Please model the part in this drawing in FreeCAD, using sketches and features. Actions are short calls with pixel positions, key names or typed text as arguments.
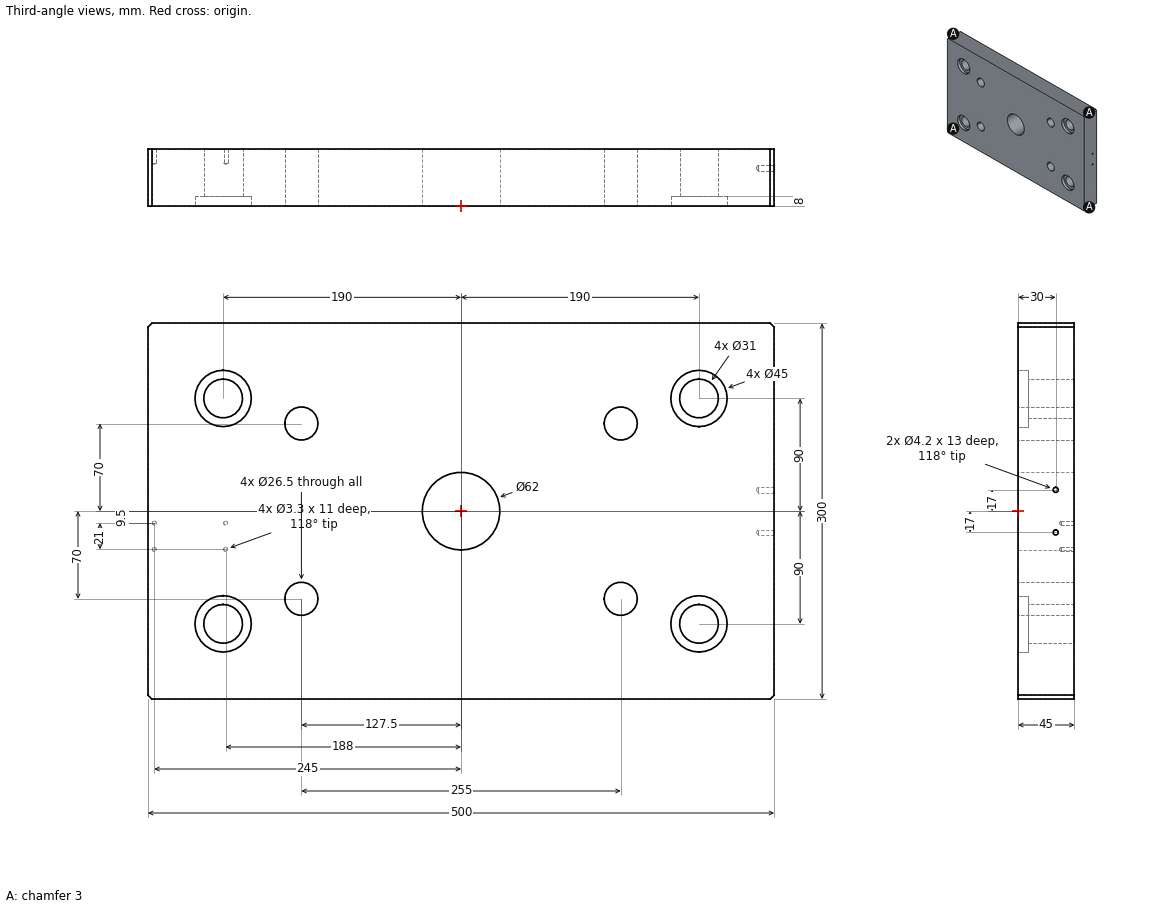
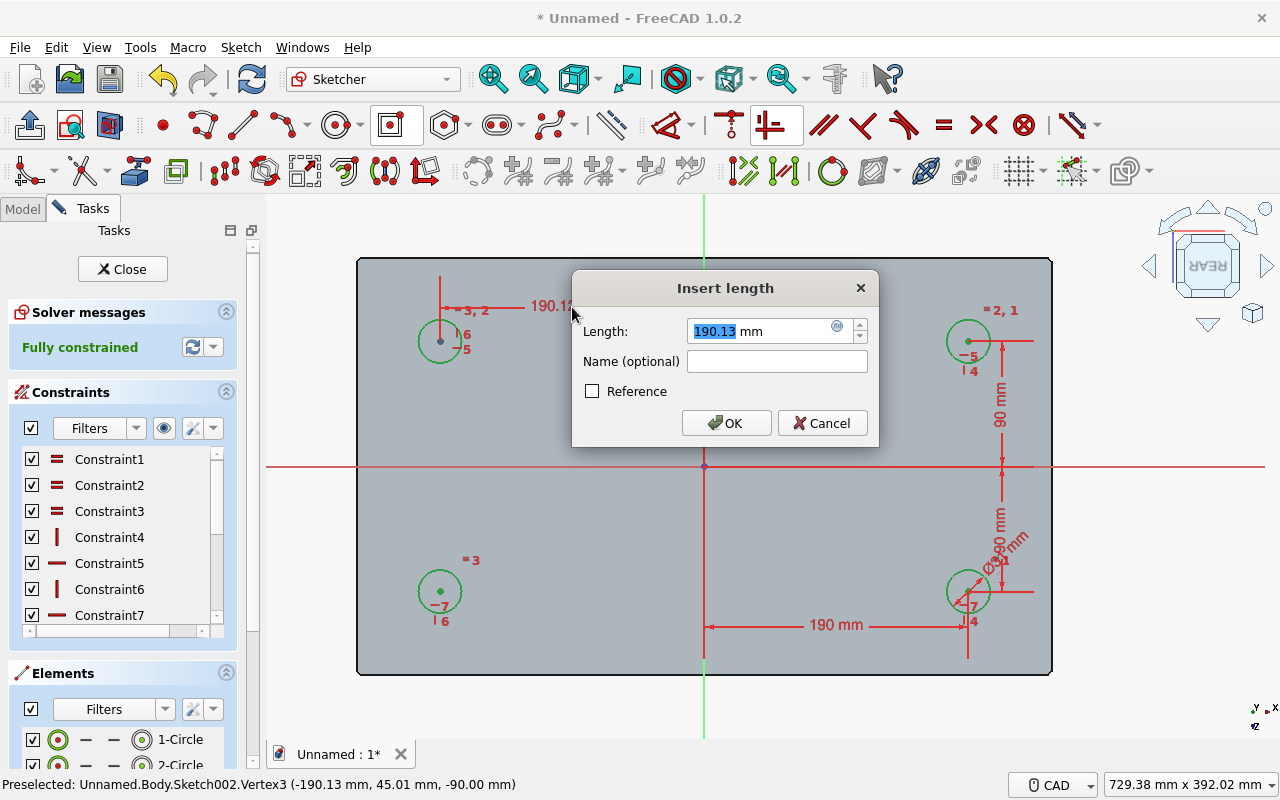
text(190)
key(Return)
key(Escape)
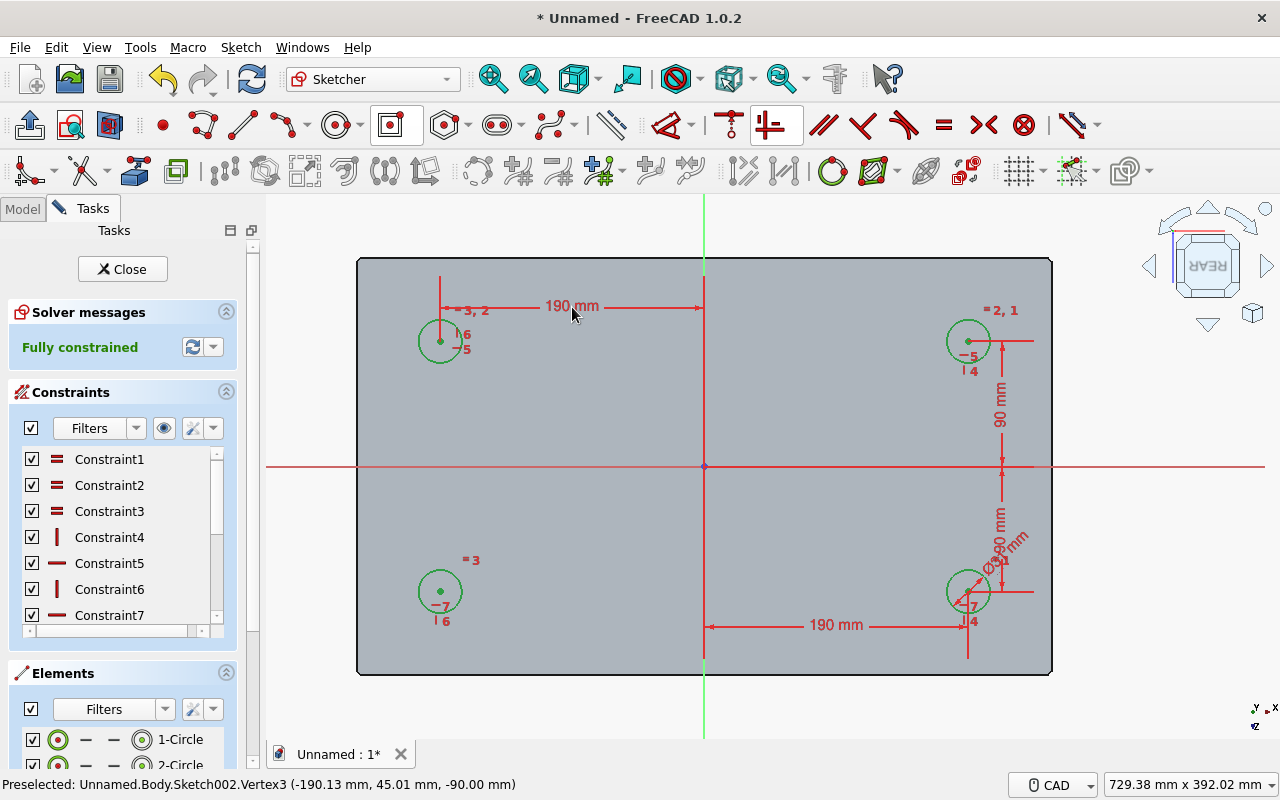
click(123, 269)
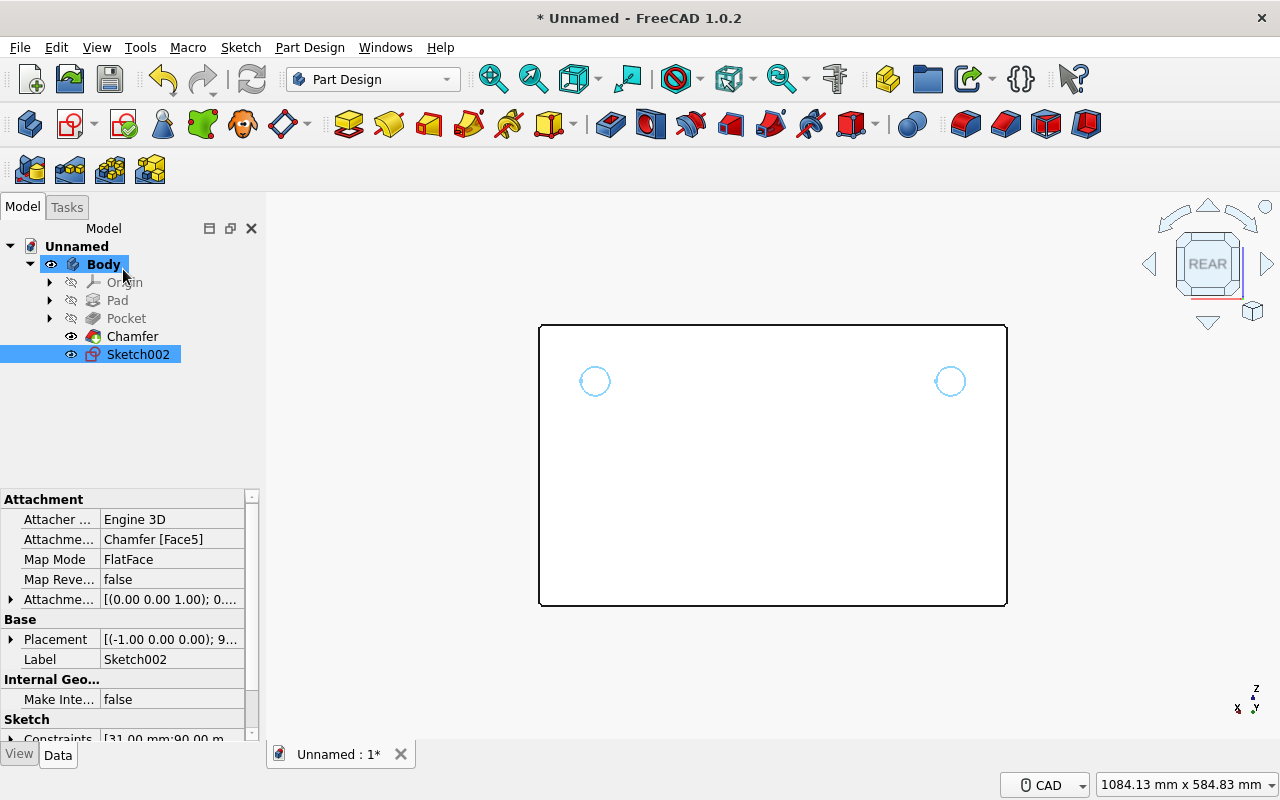
click(612, 124)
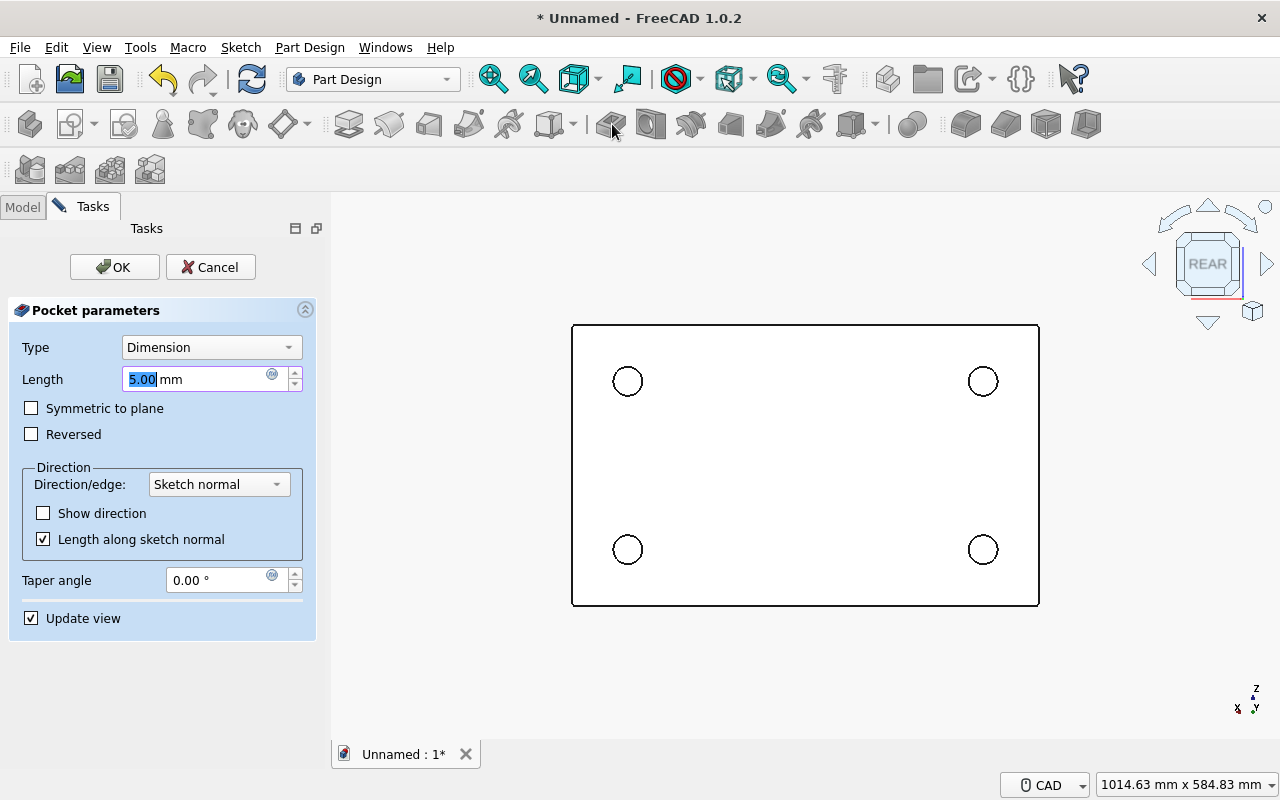
click(212, 348)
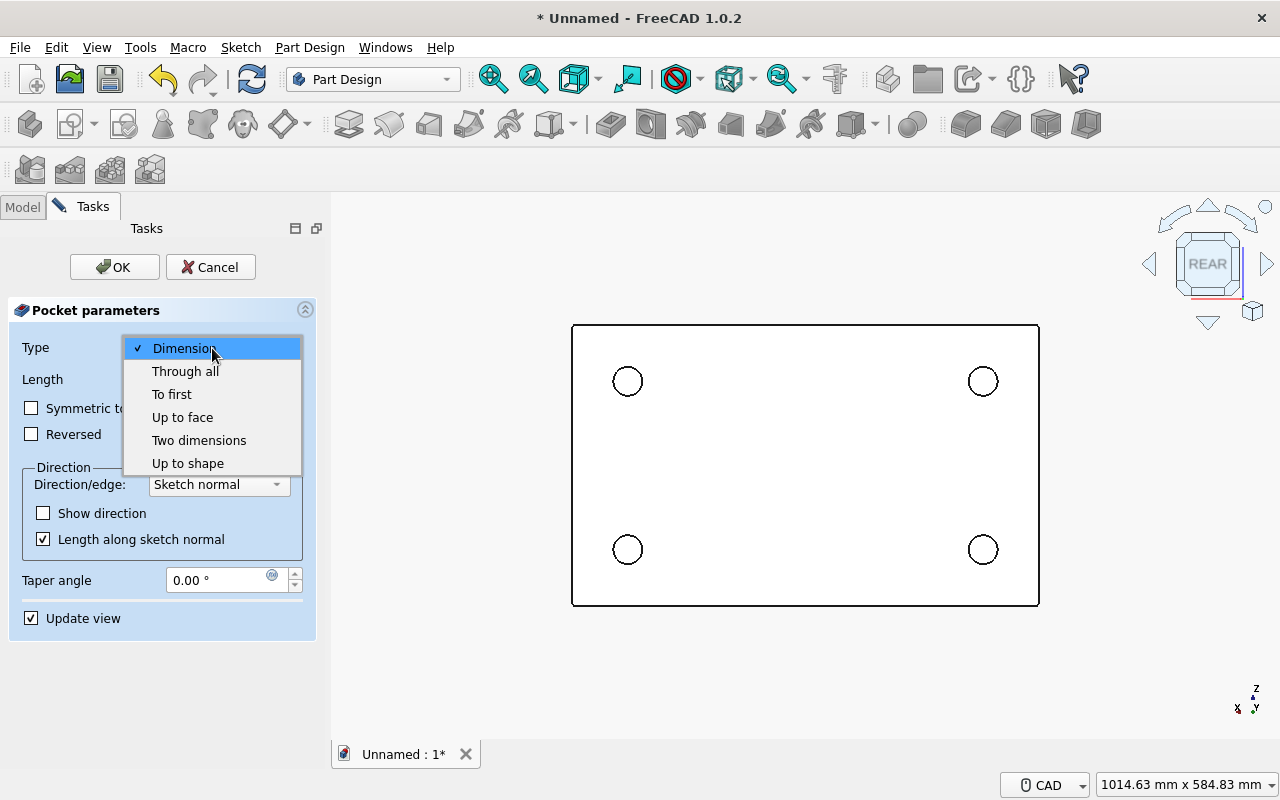
click(212, 372)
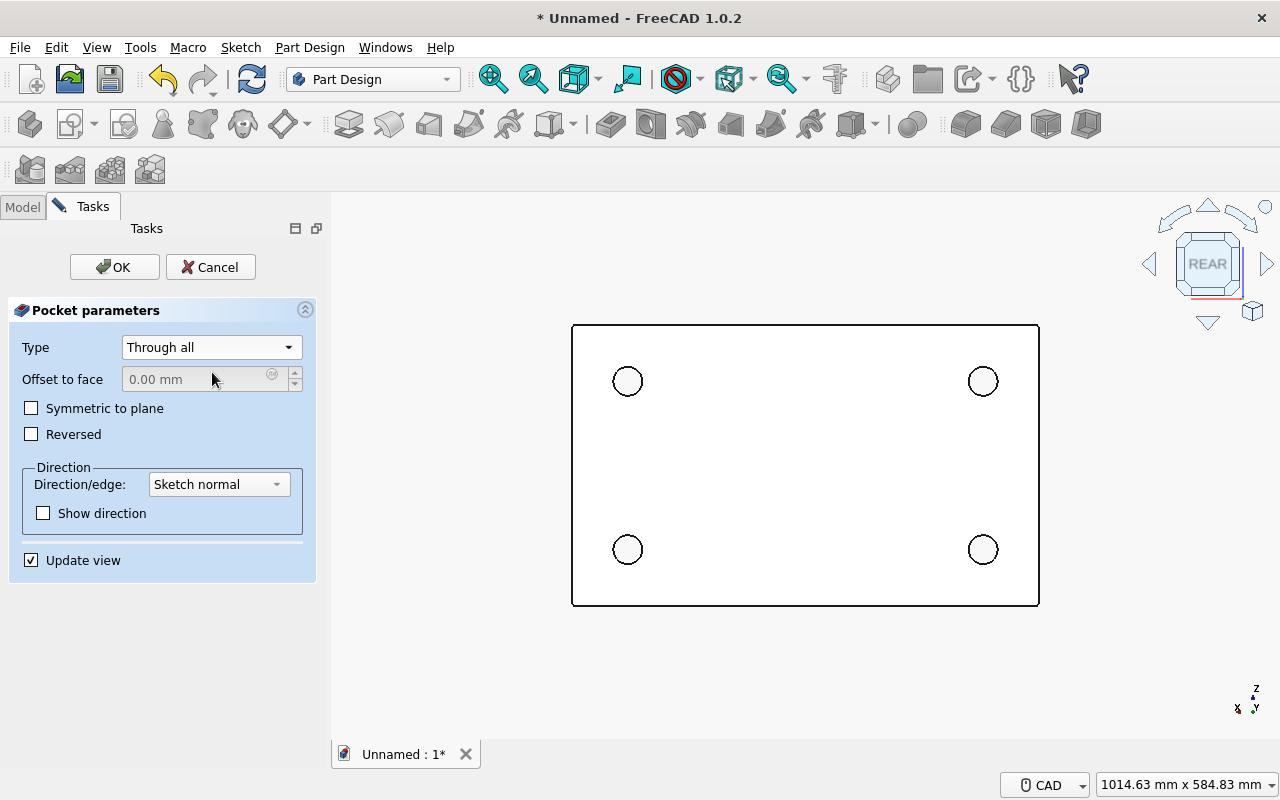
click(115, 267)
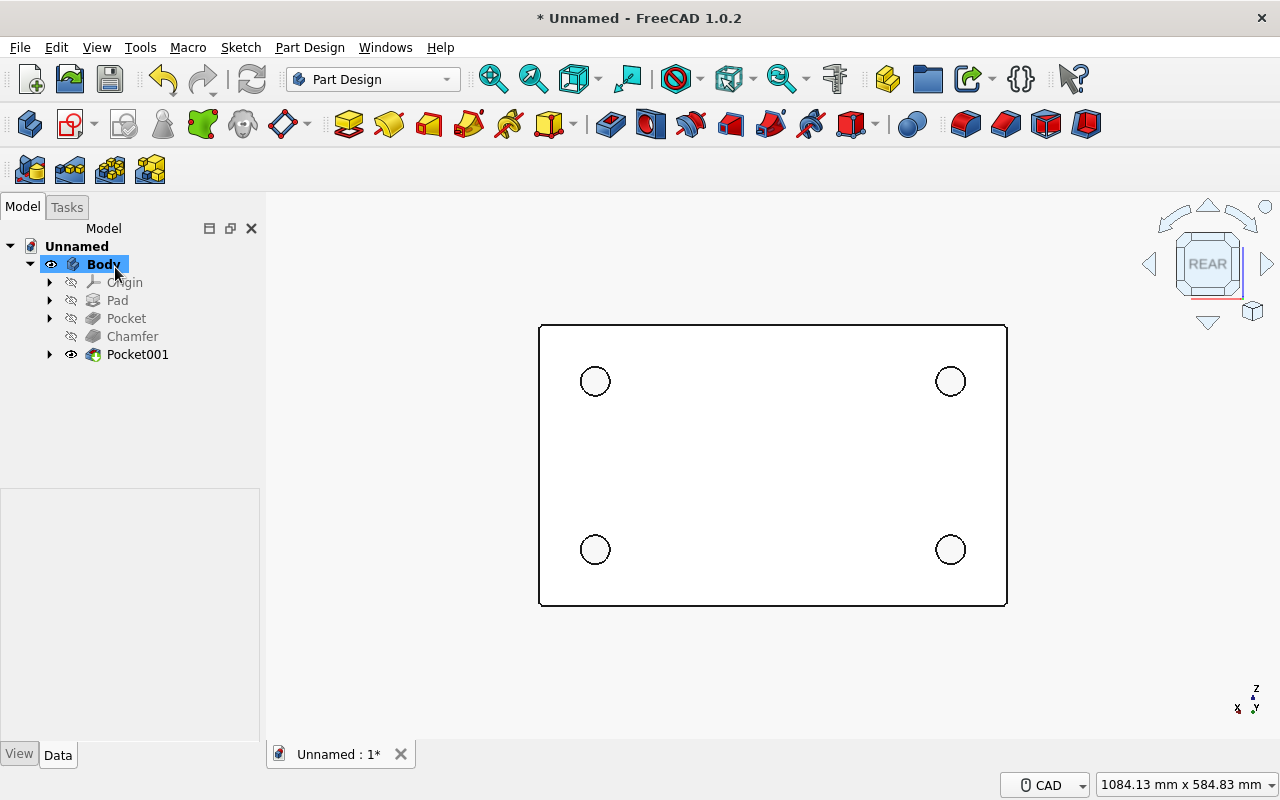
click(70, 124)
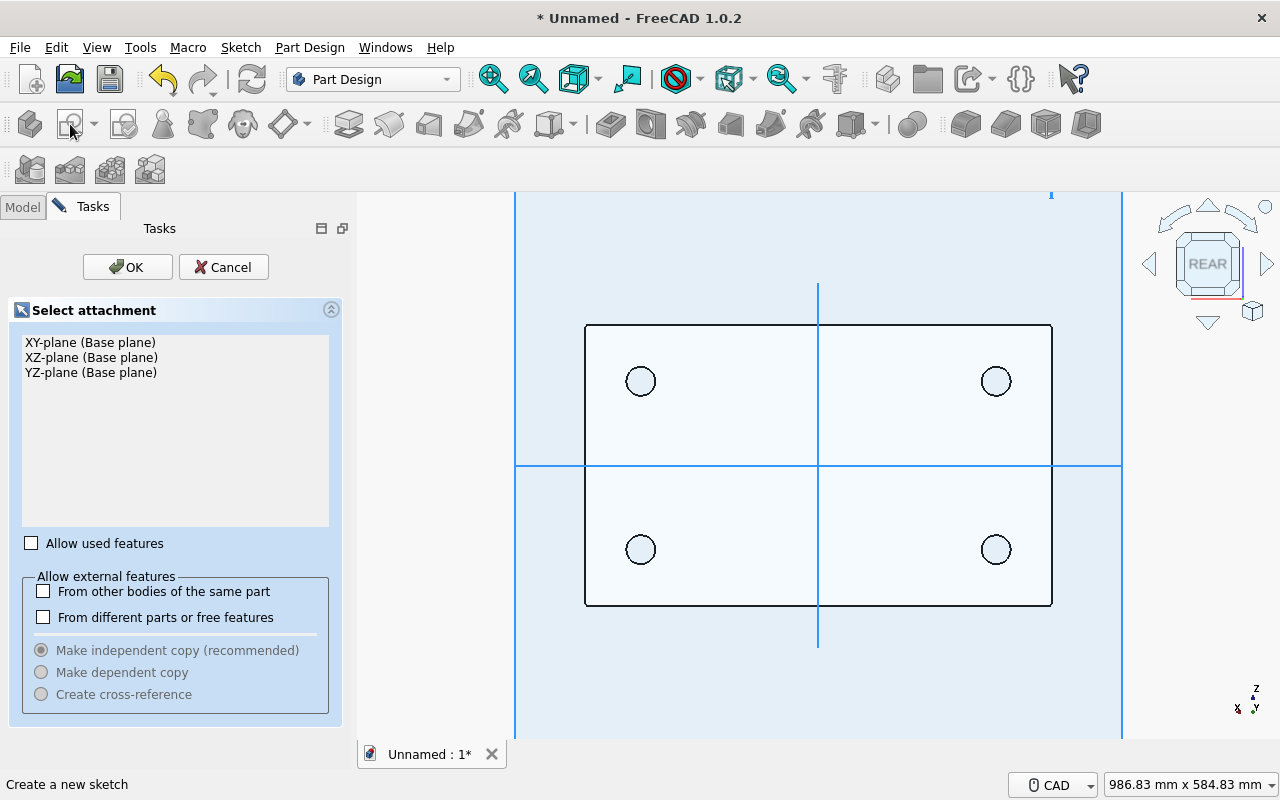
click(82, 358)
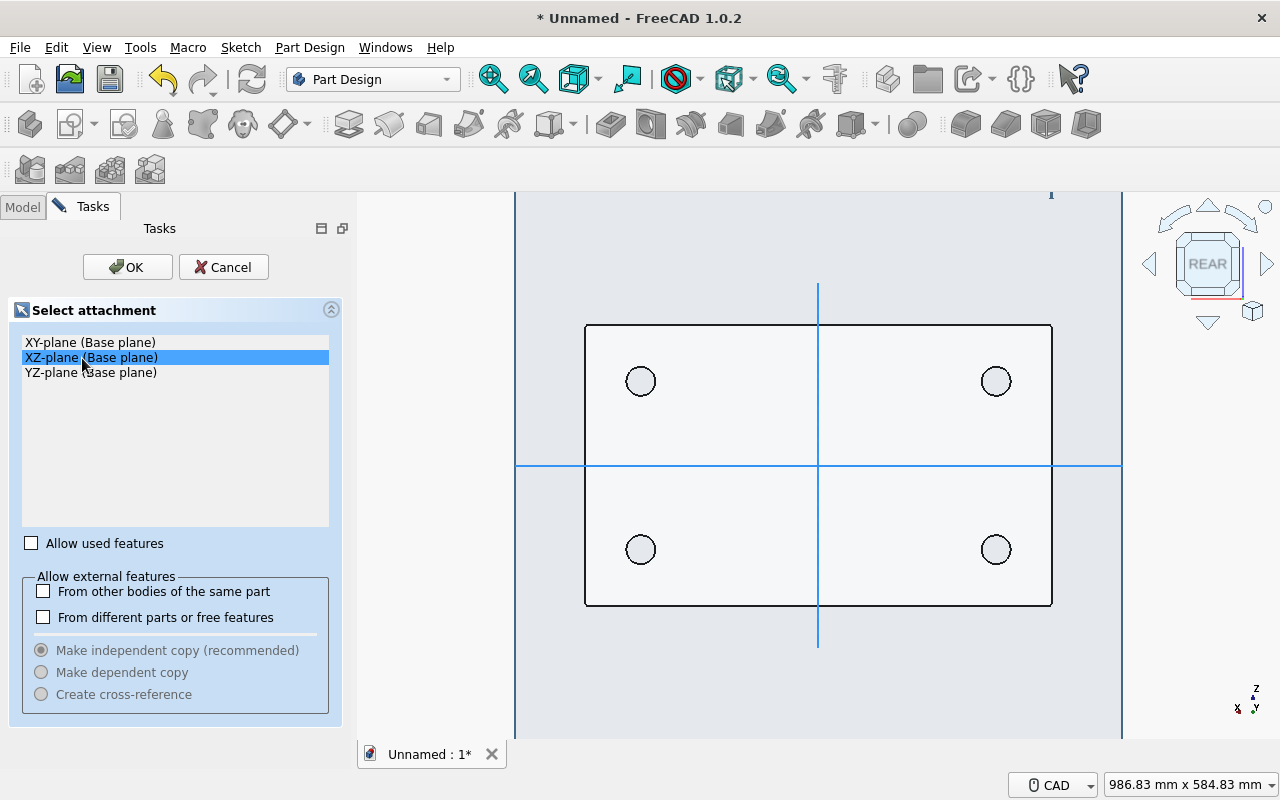
click(128, 267)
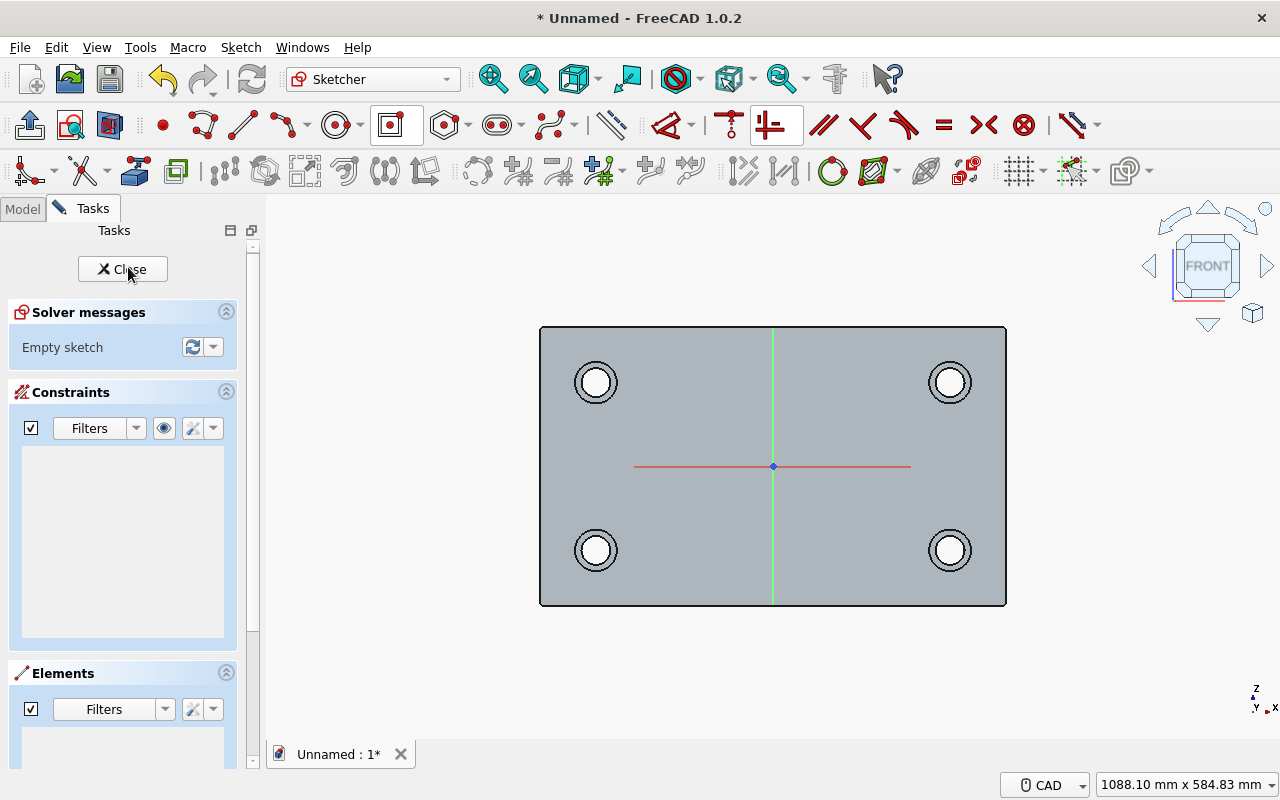
scroll(787, 467, up, 9)